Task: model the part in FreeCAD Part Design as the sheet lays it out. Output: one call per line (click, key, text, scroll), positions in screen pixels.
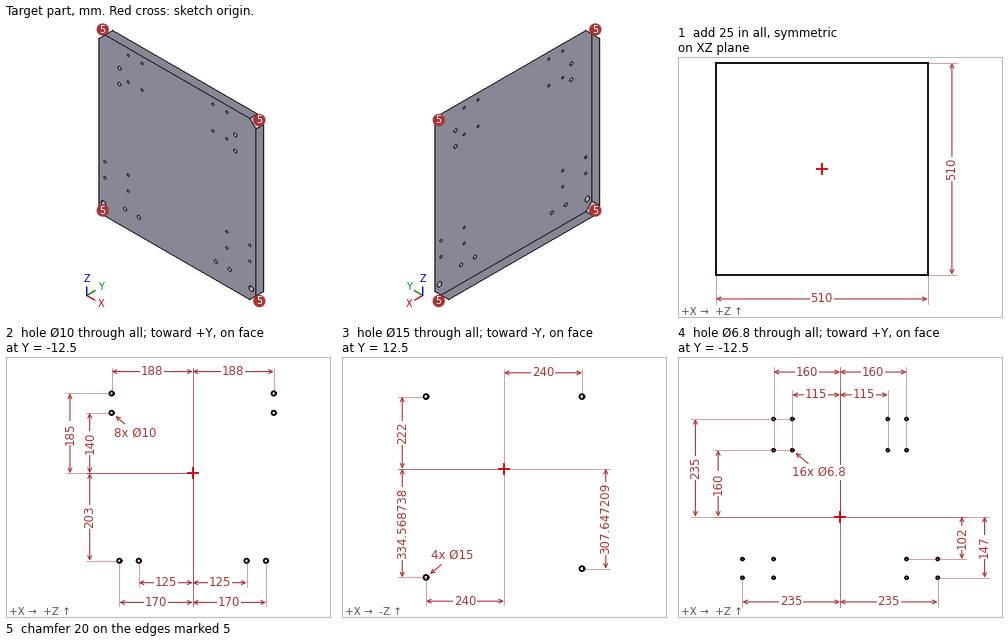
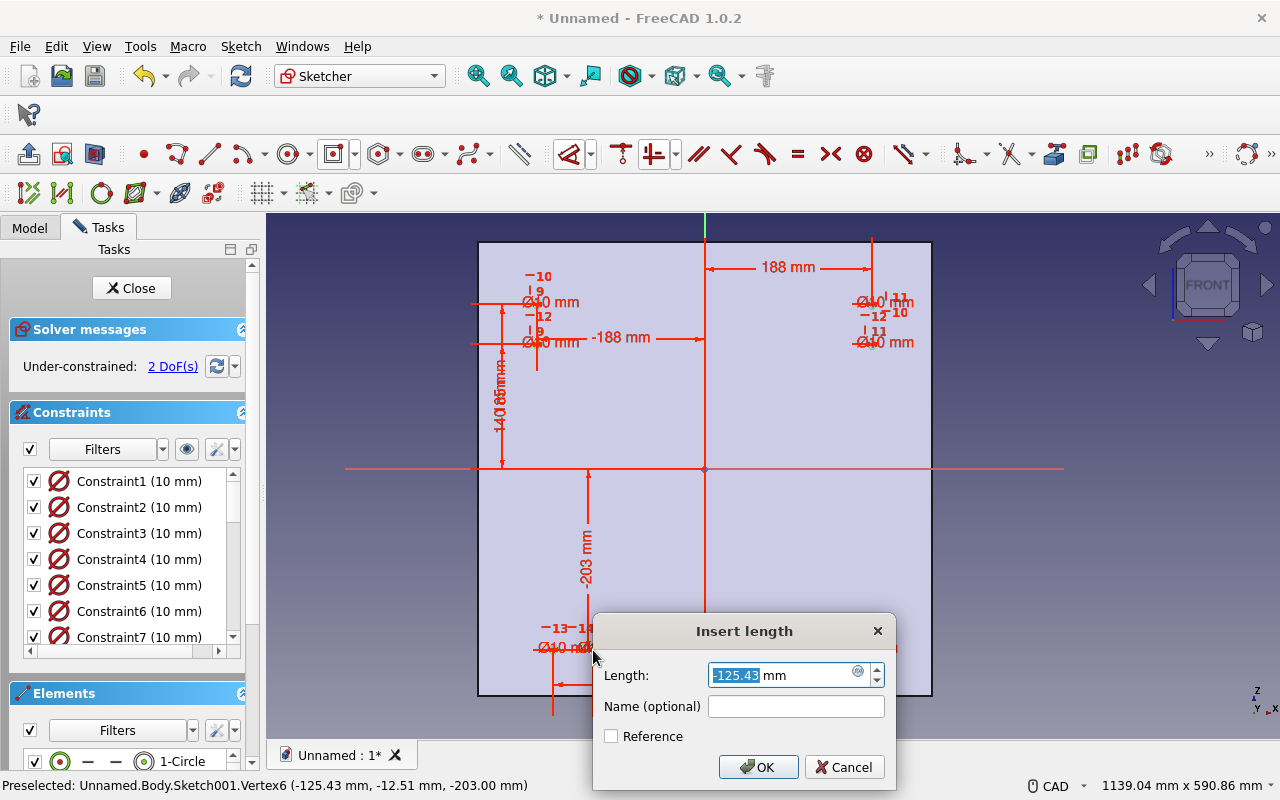
text(-125)
key(Return)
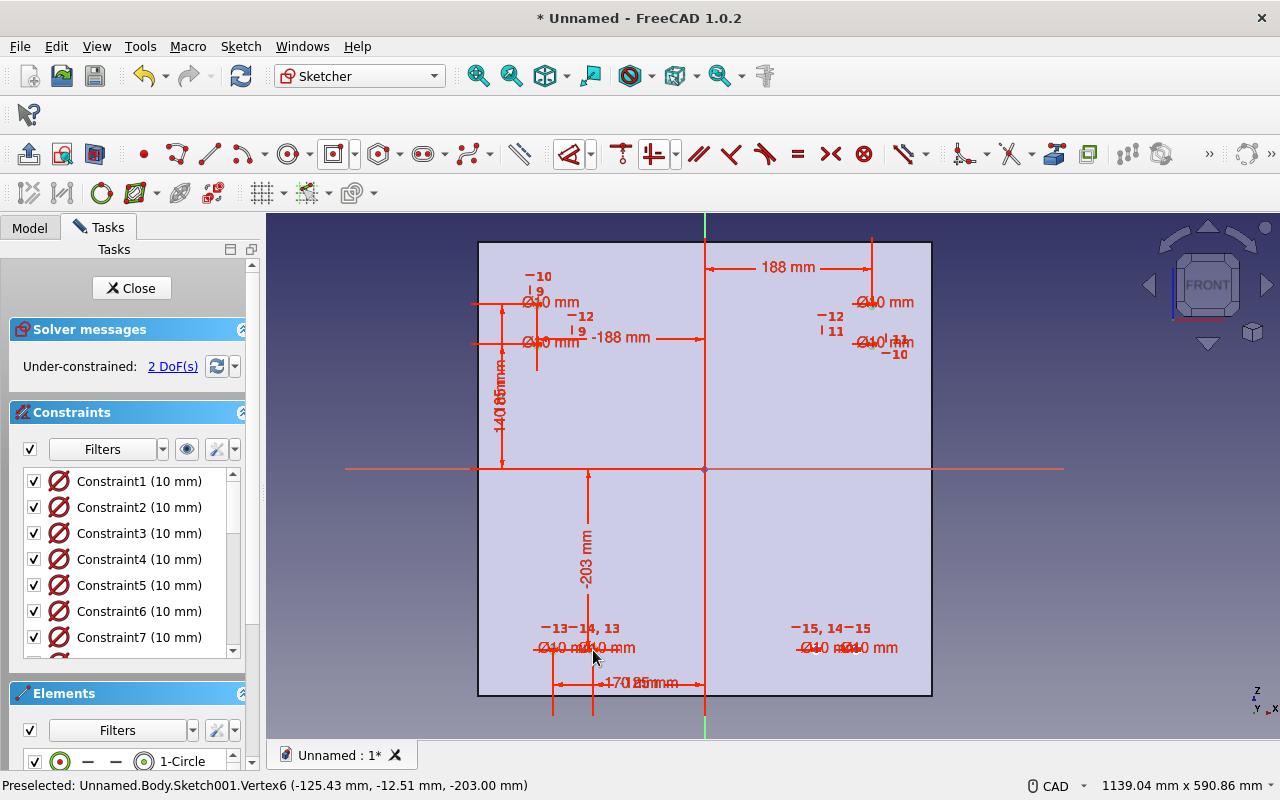
click(816, 650)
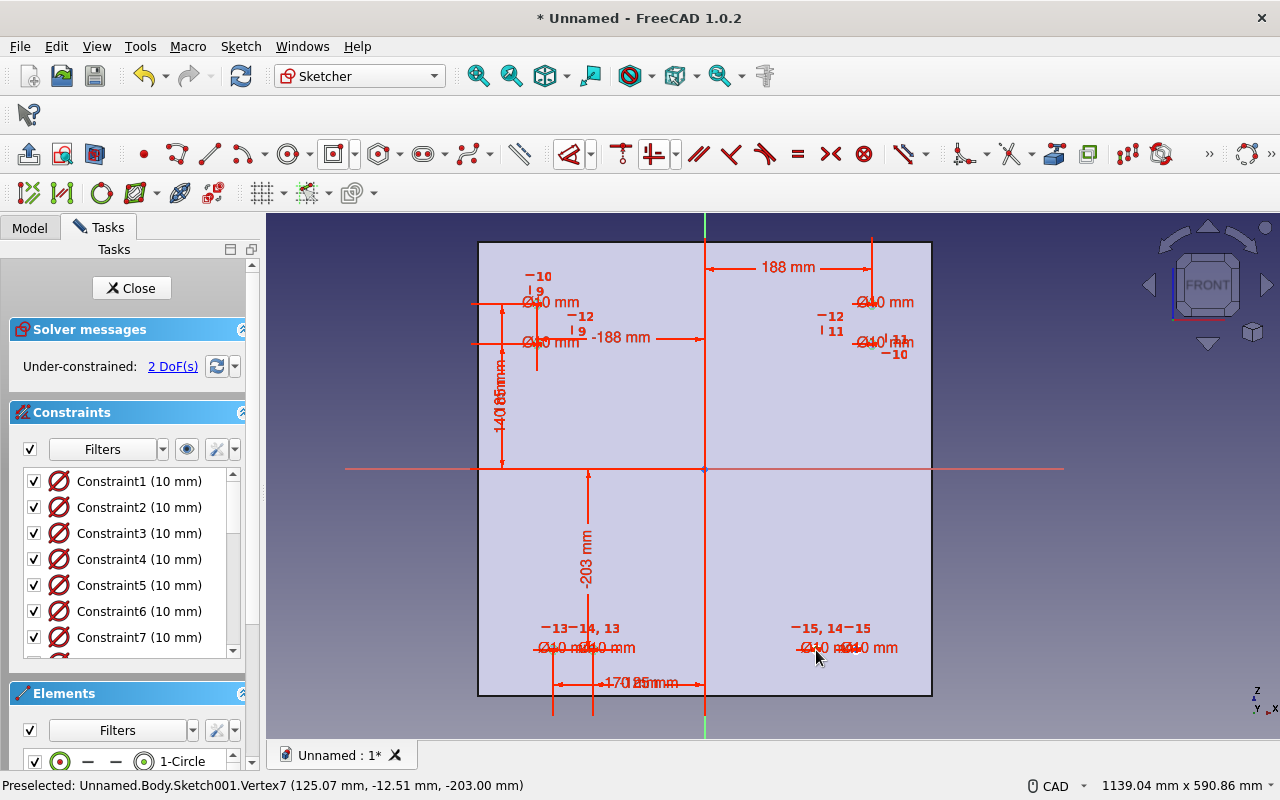
key(l)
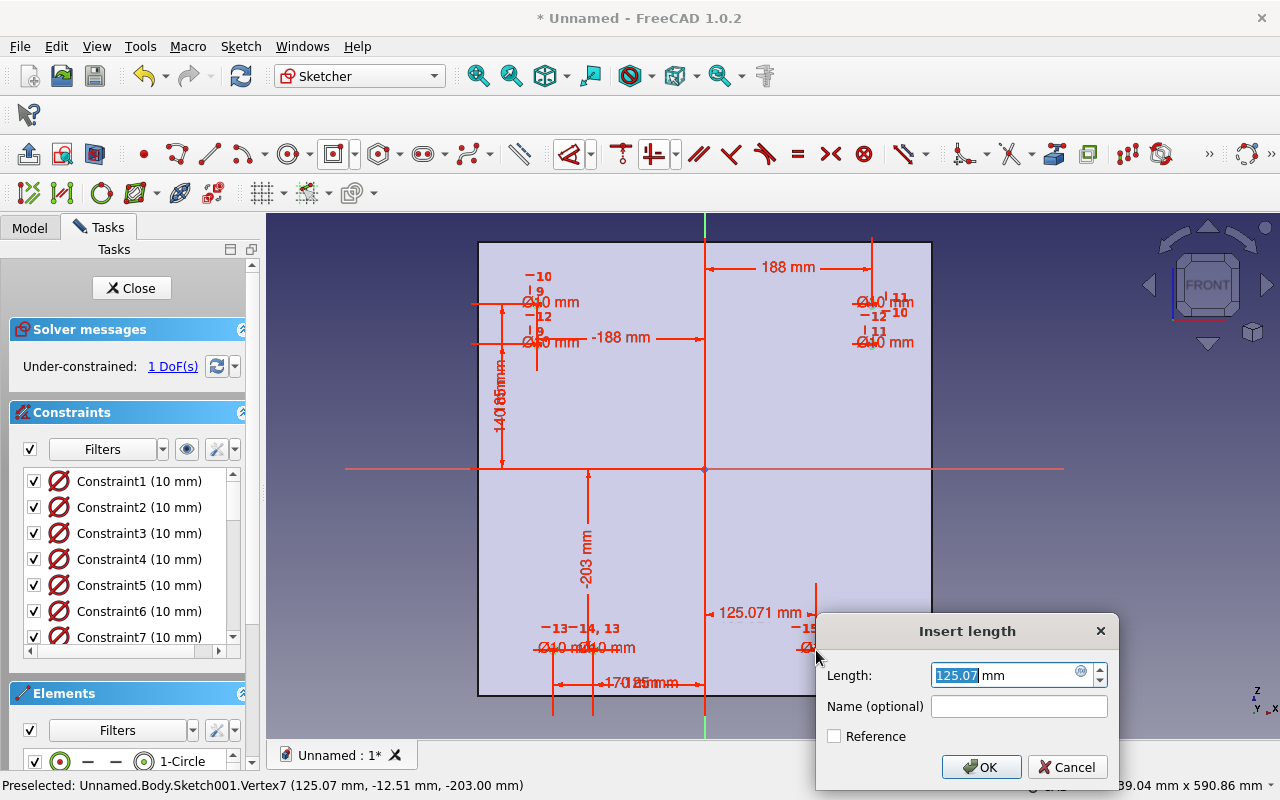
text(125)
key(Return)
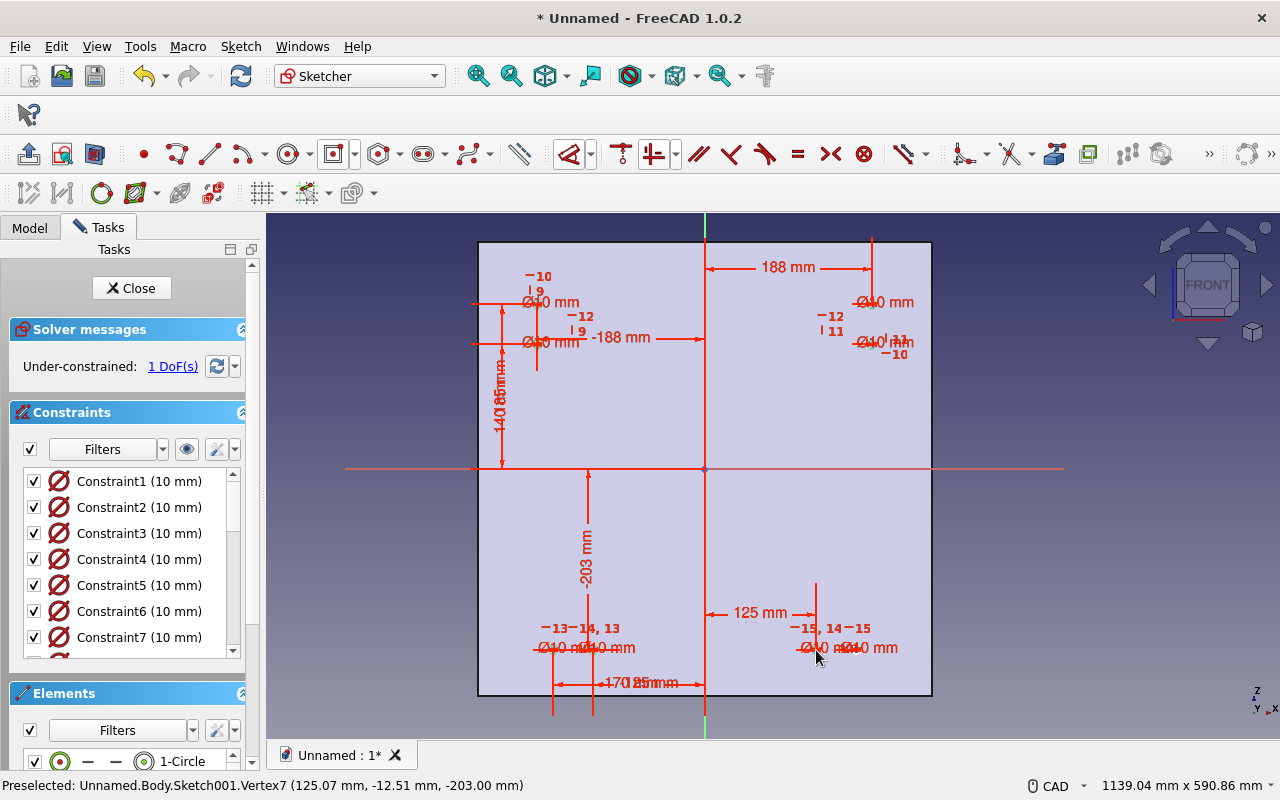
click(856, 650)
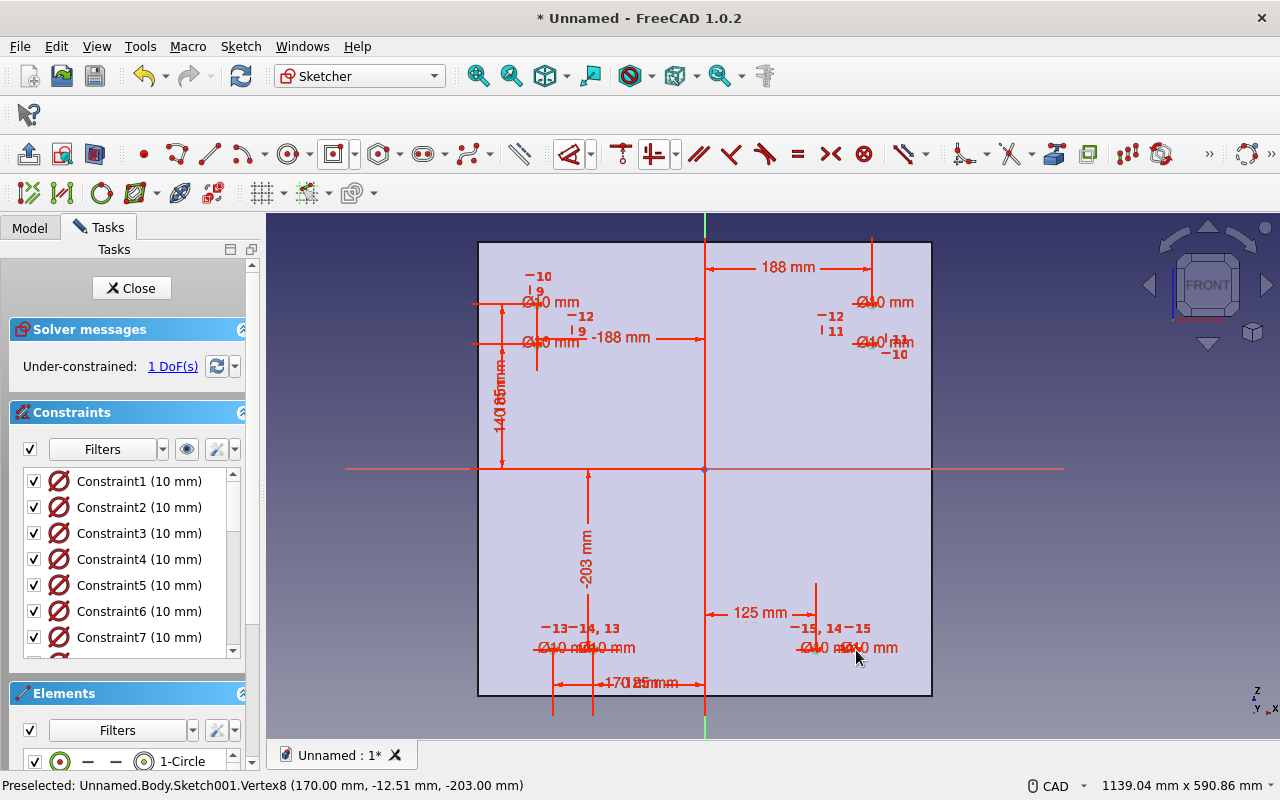
key(l)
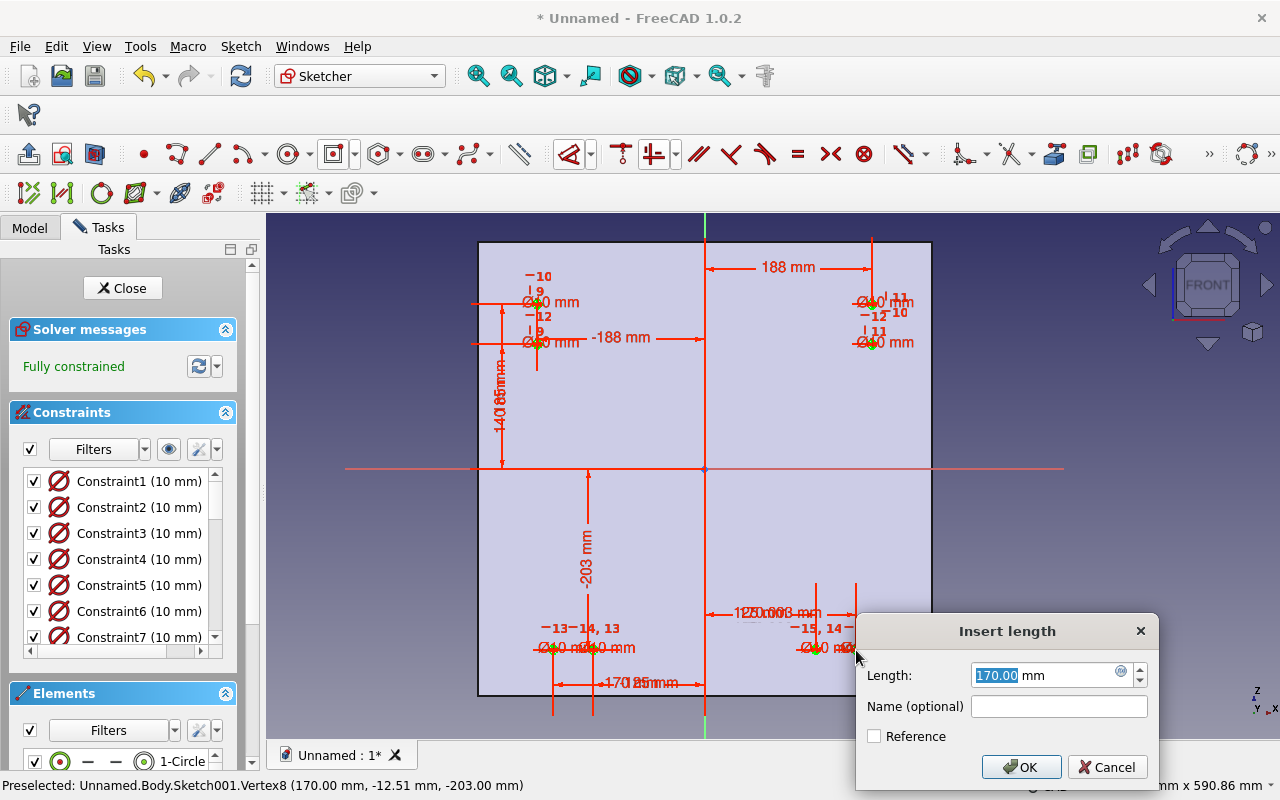
text(170)
key(Return)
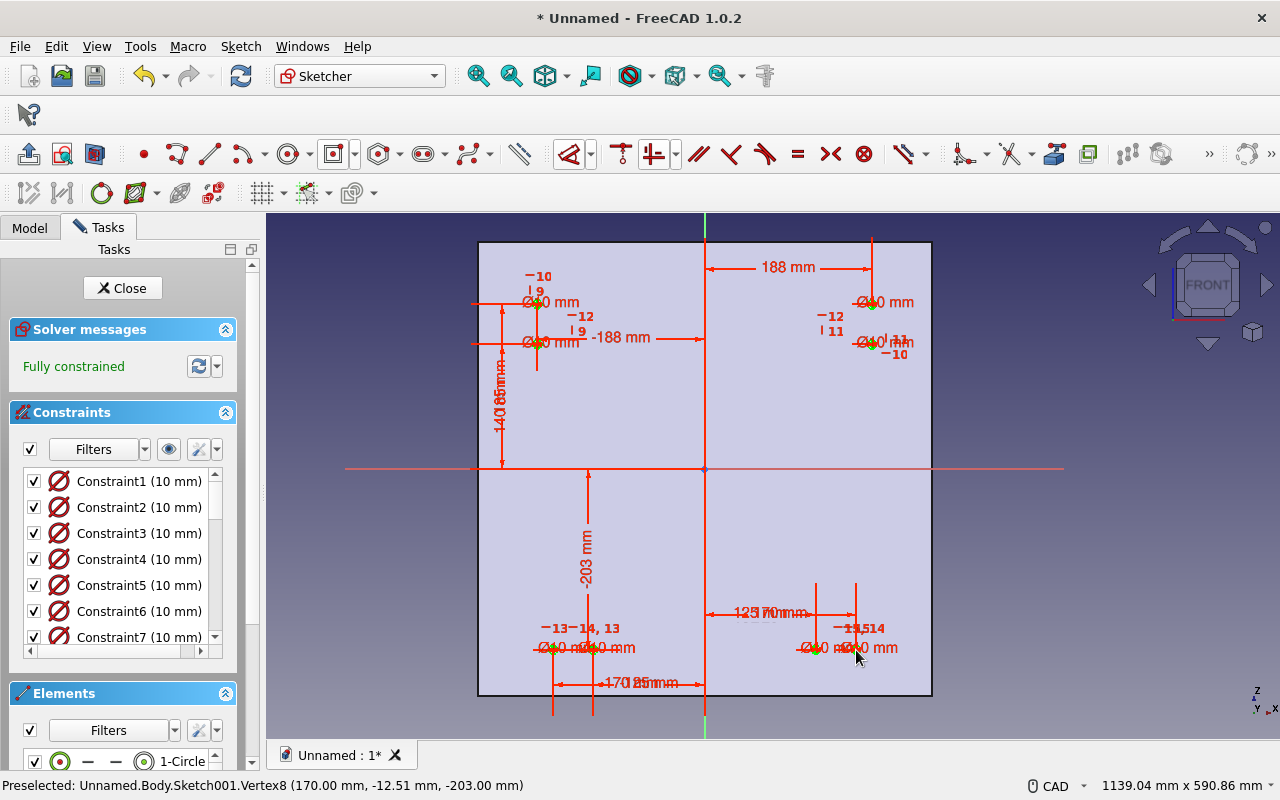
click(123, 288)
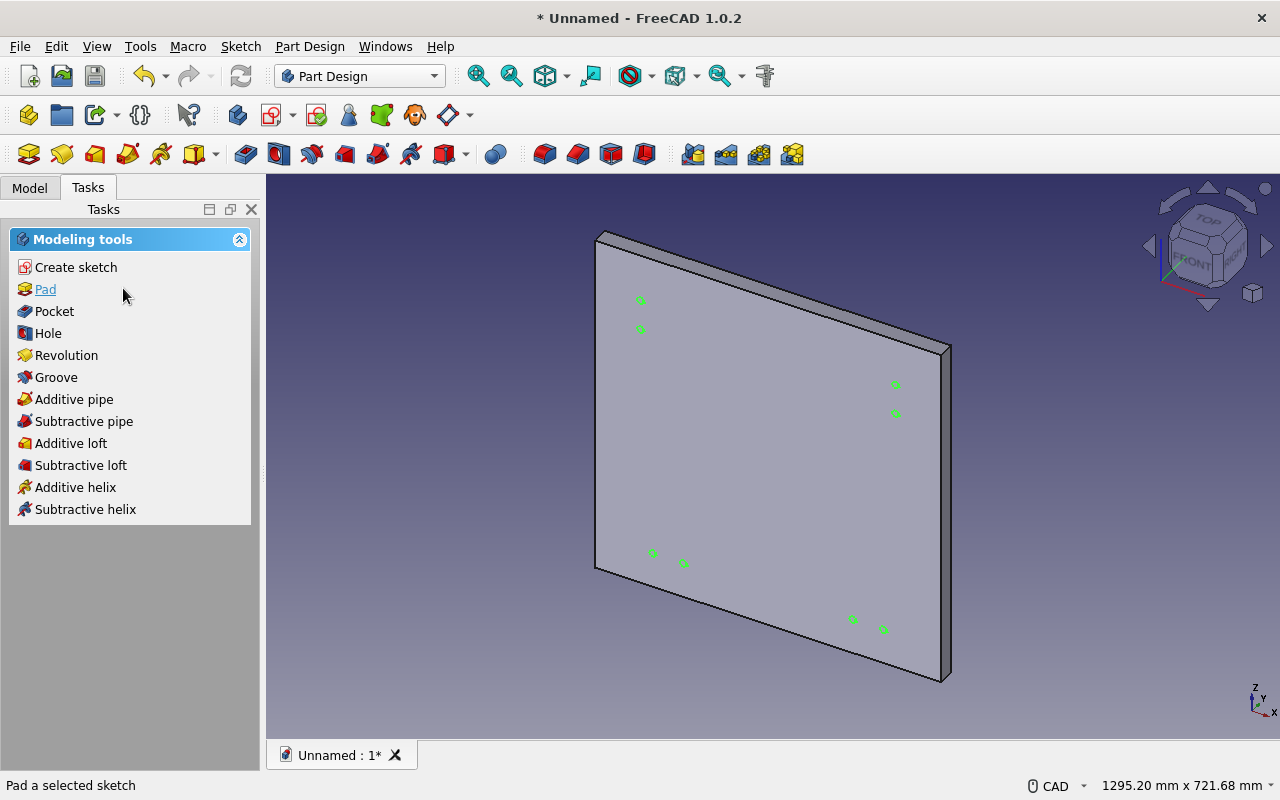
click(279, 154)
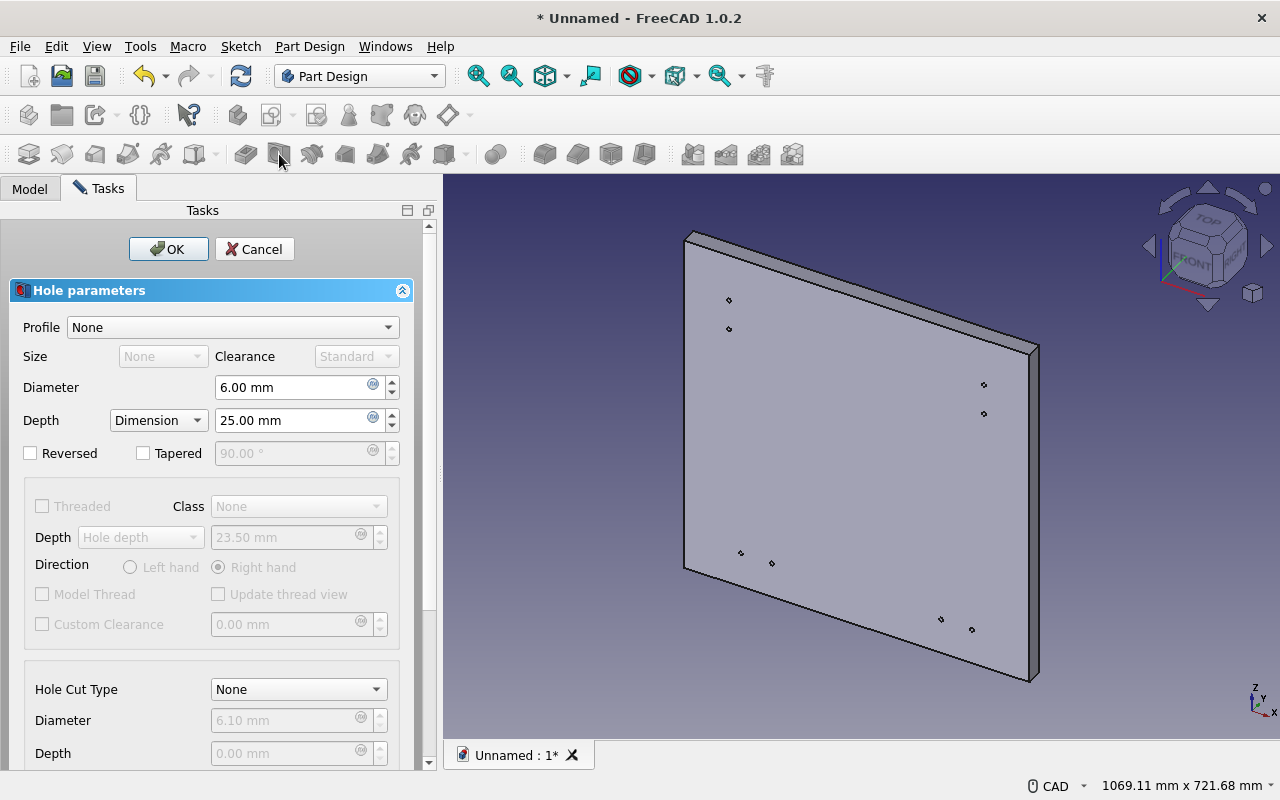
triple_click(300, 388)